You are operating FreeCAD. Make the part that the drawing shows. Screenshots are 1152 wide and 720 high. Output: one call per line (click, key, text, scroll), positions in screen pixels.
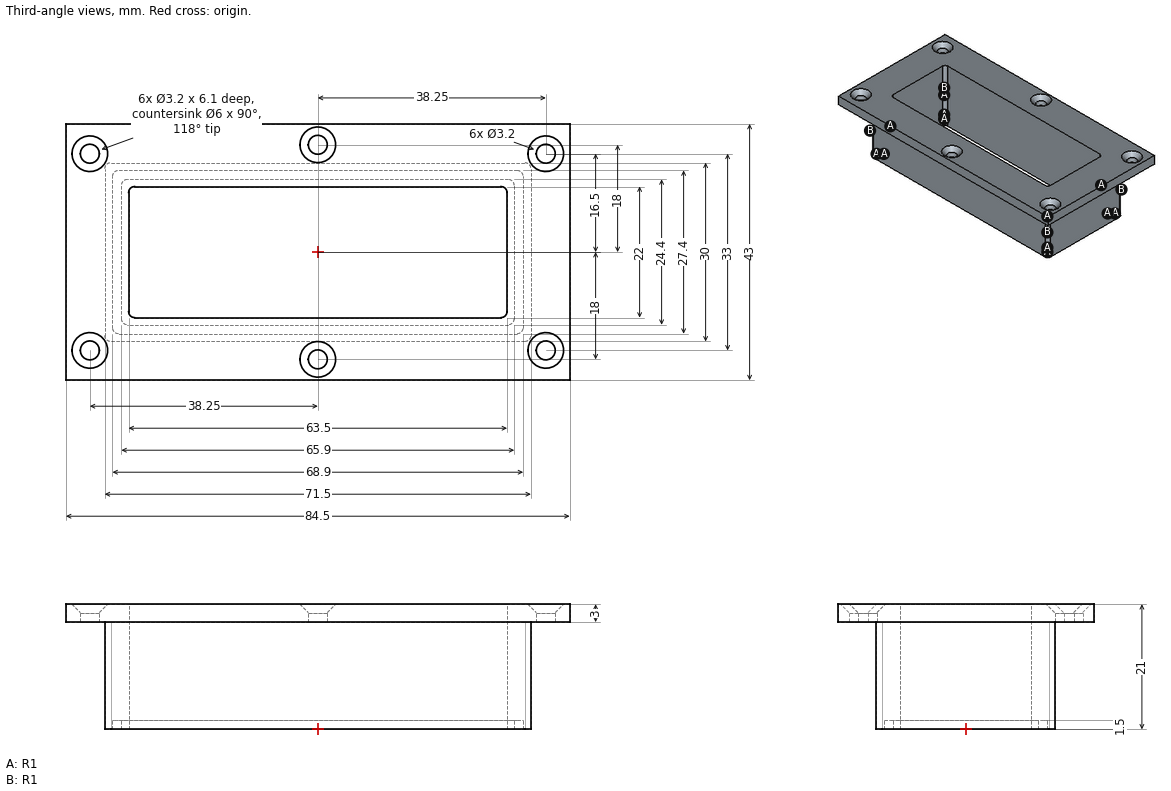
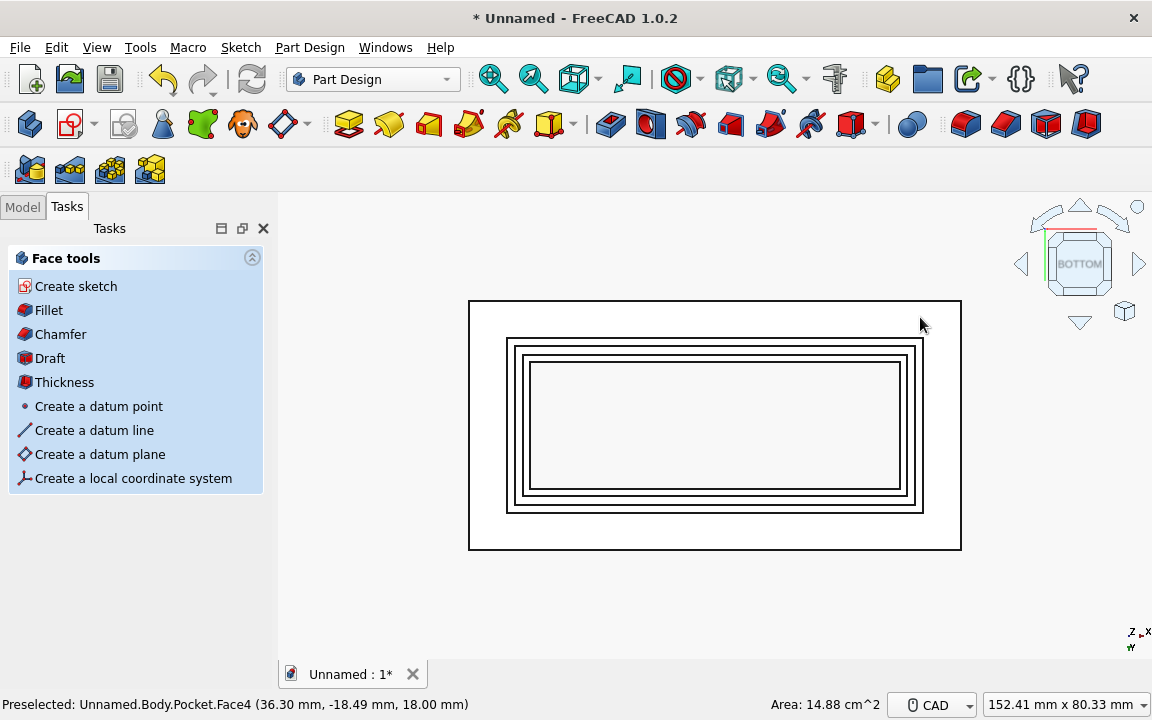
click(70, 124)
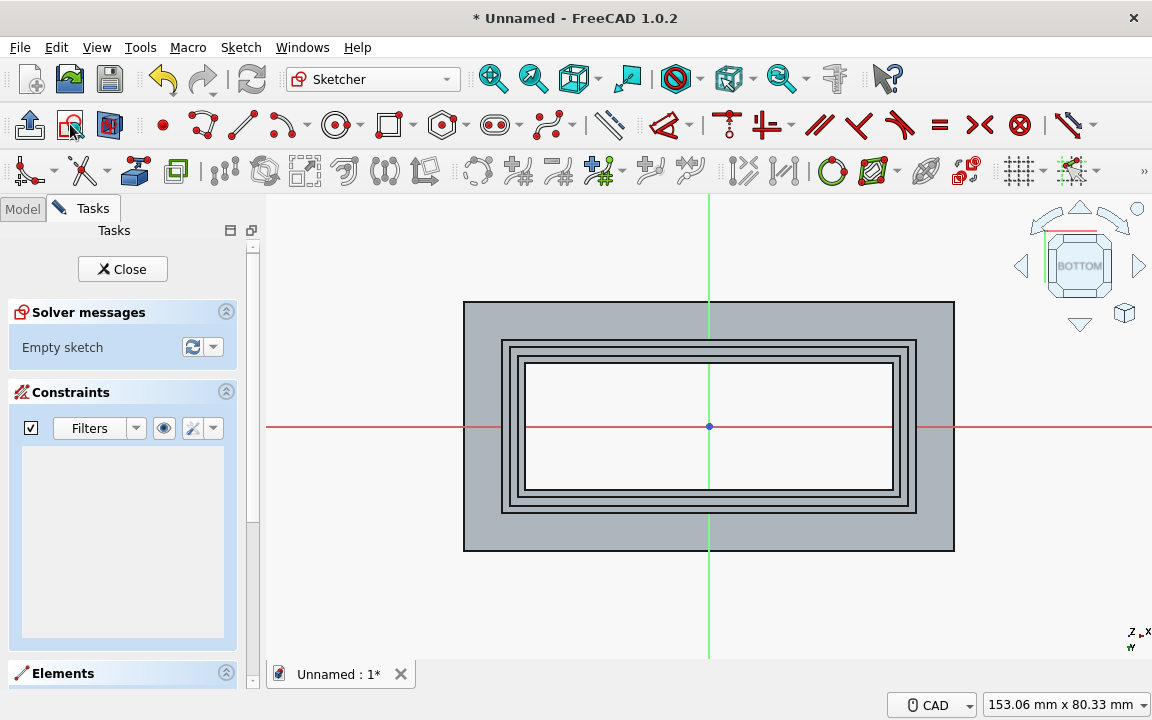
click(336, 126)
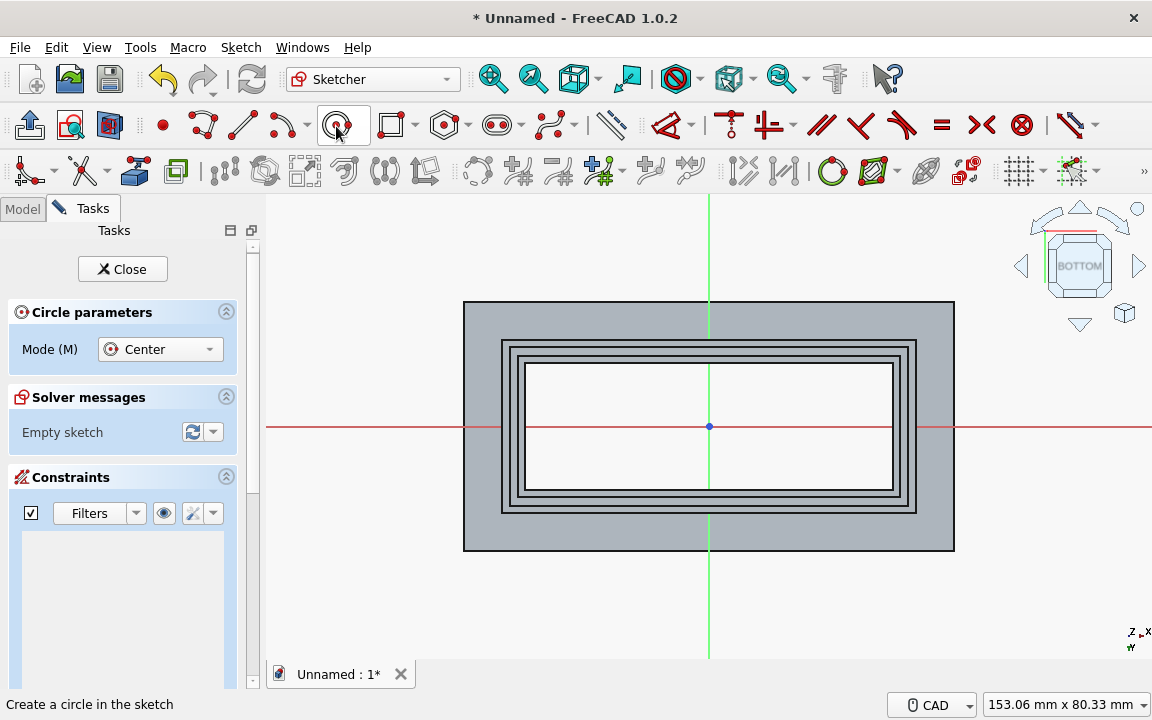
scroll(930, 522, up, 5)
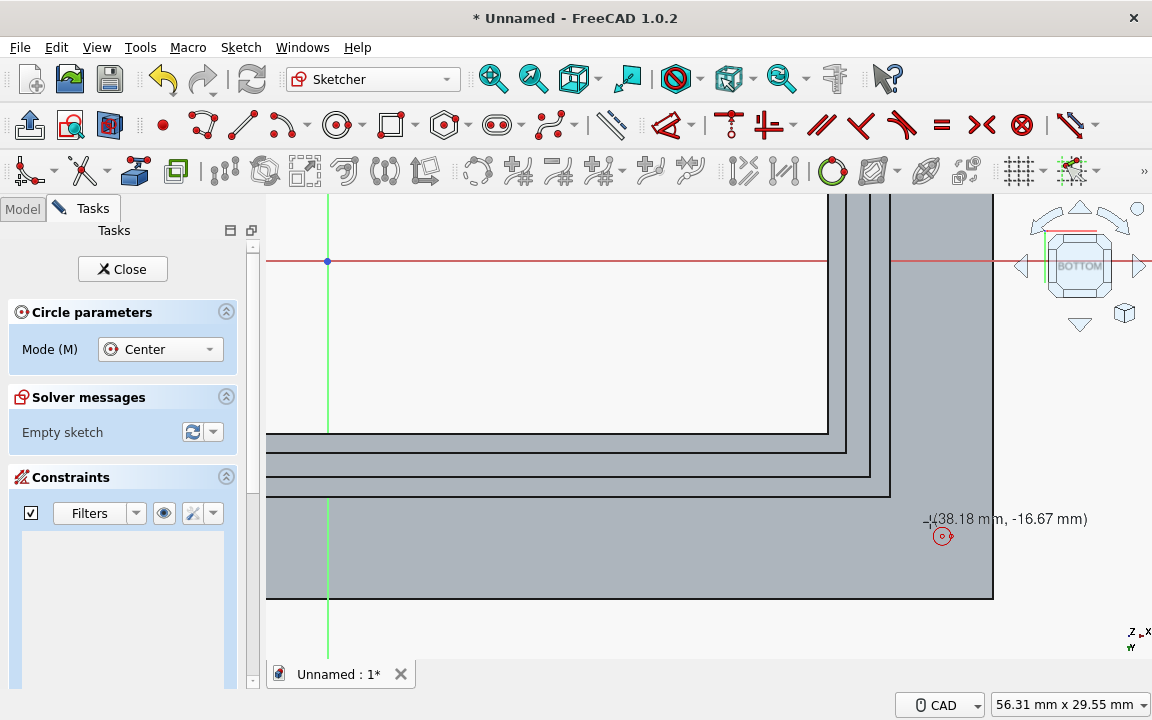
click(930, 521)
click(948, 503)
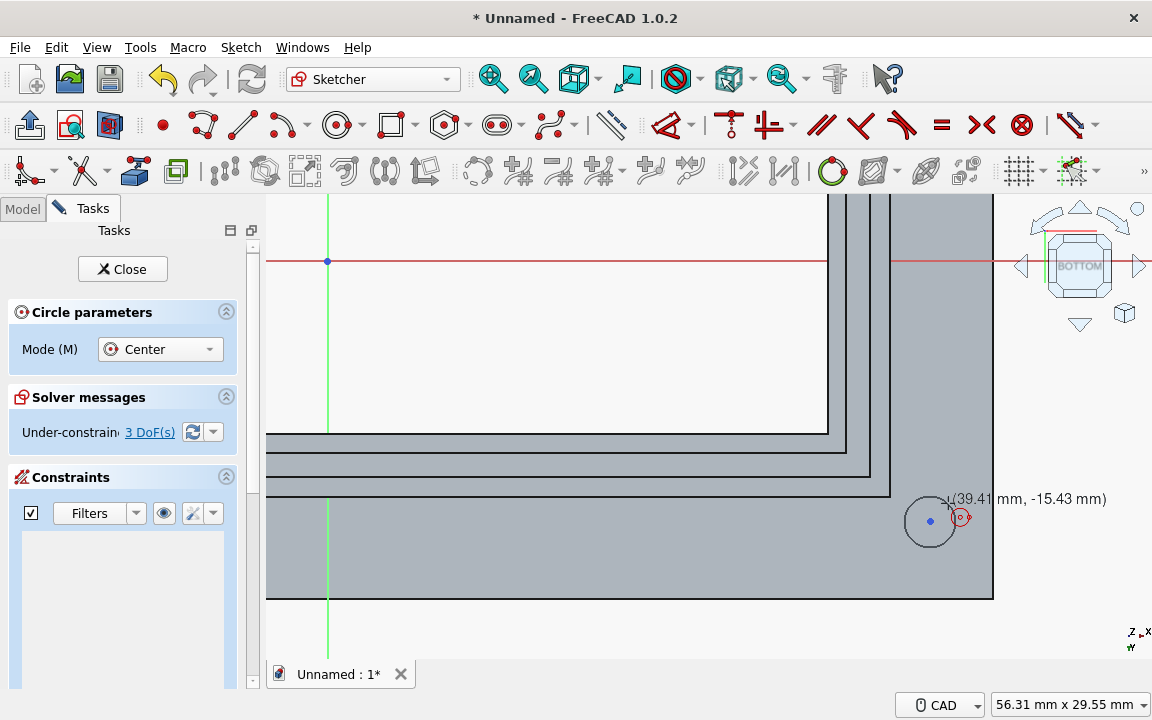
scroll(822, 523, down, 5)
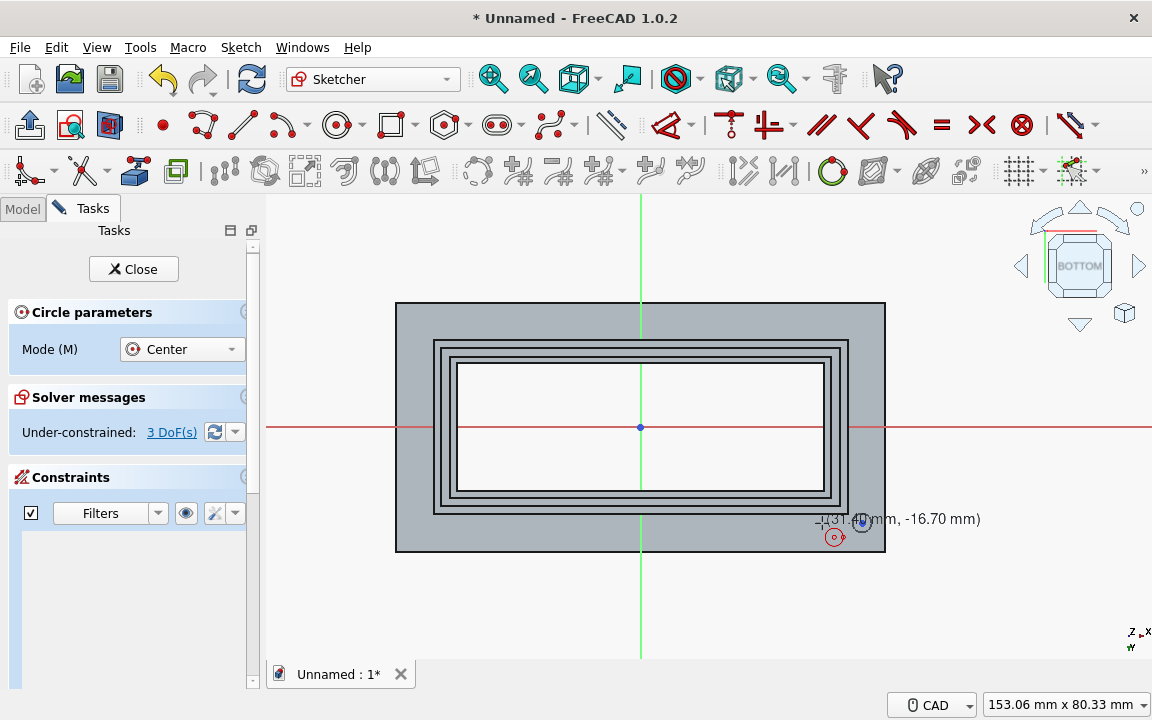
scroll(862, 332, up, 5)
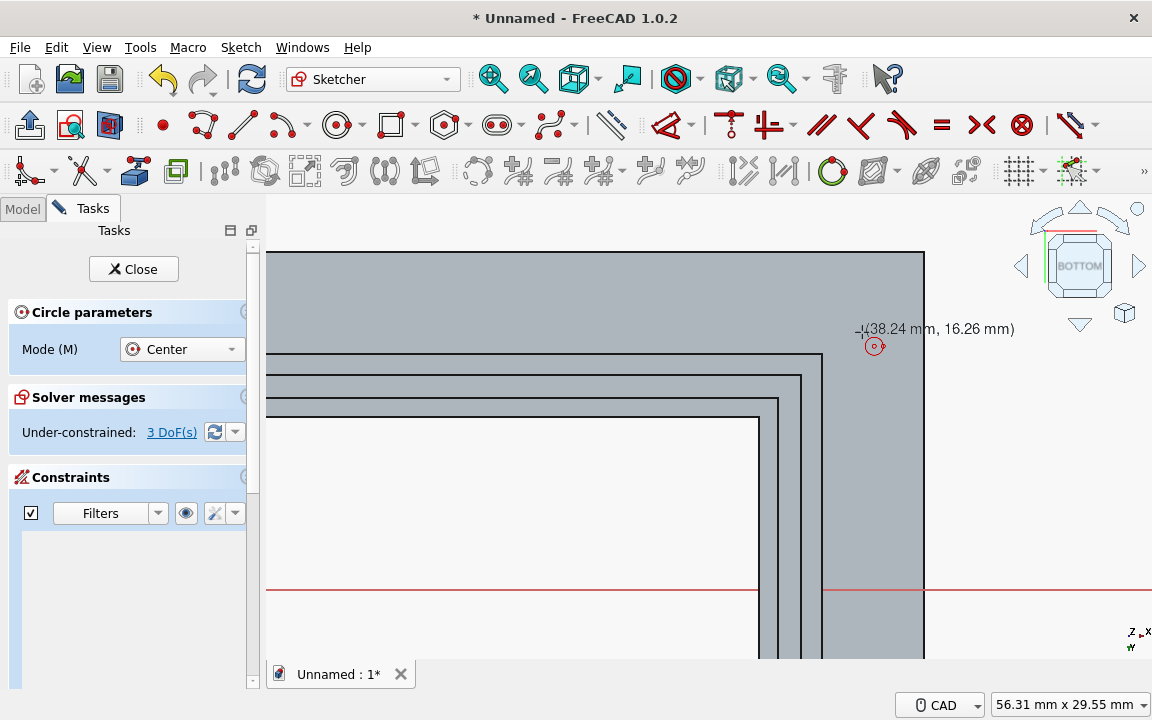
click(861, 330)
click(879, 313)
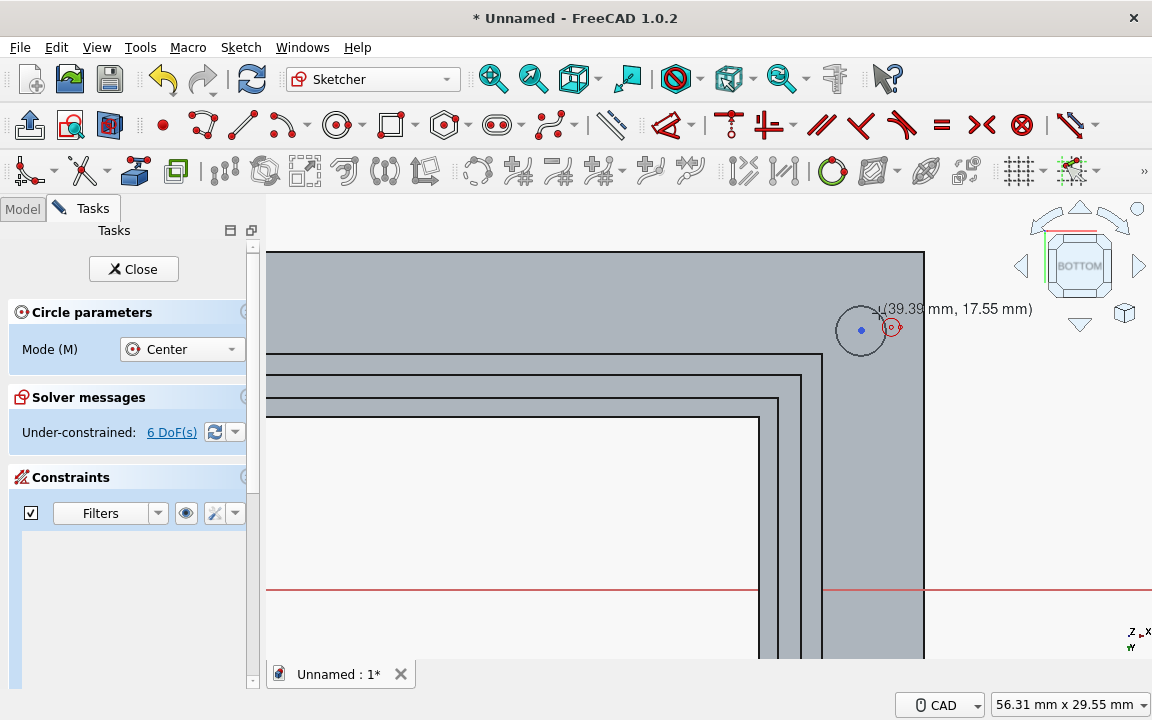
scroll(862, 331, down, 5)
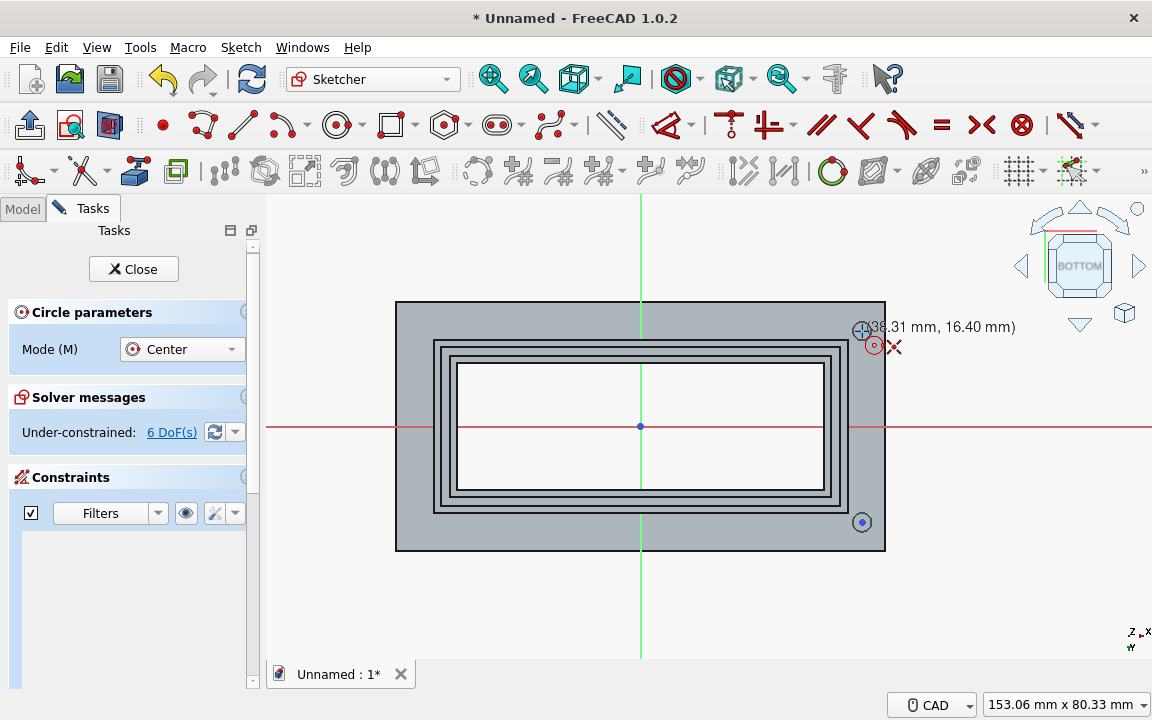
scroll(419, 331, up, 5)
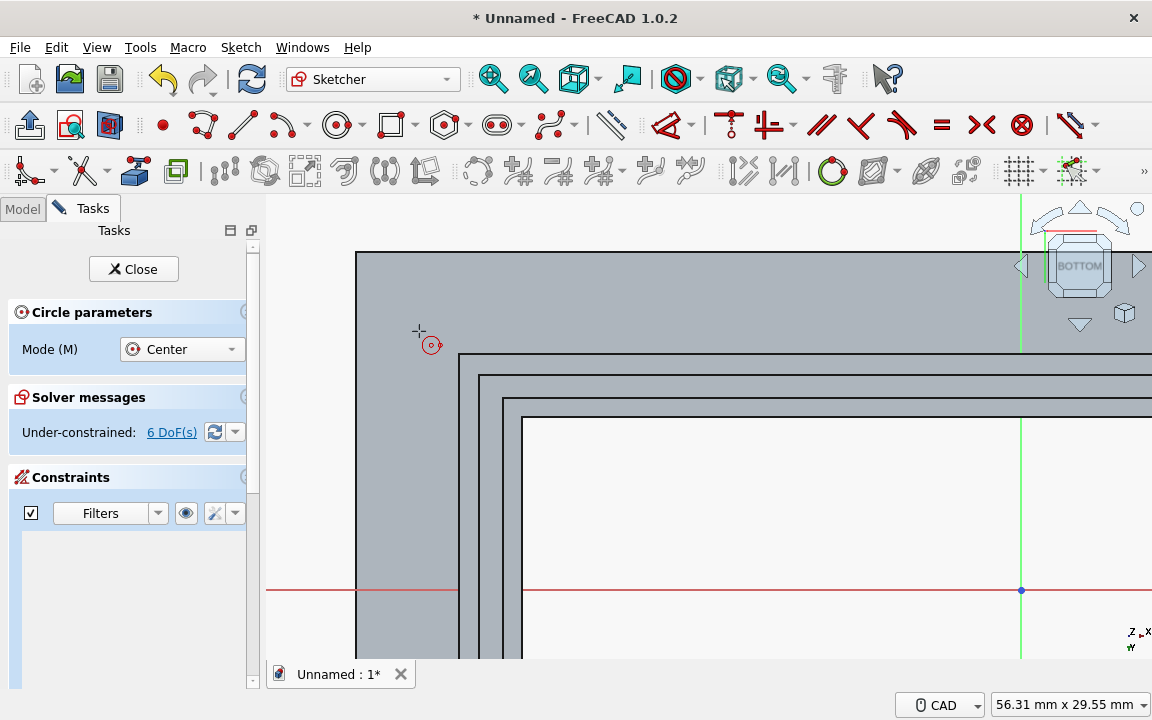
click(419, 330)
click(437, 313)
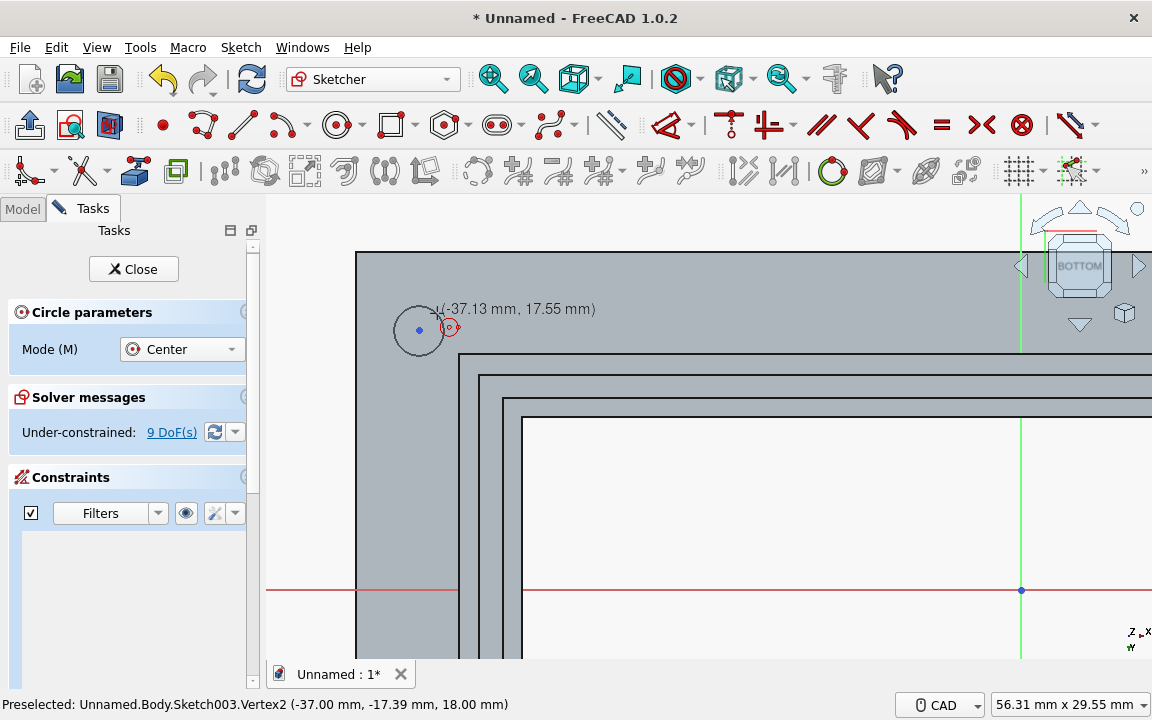
scroll(419, 331, down, 5)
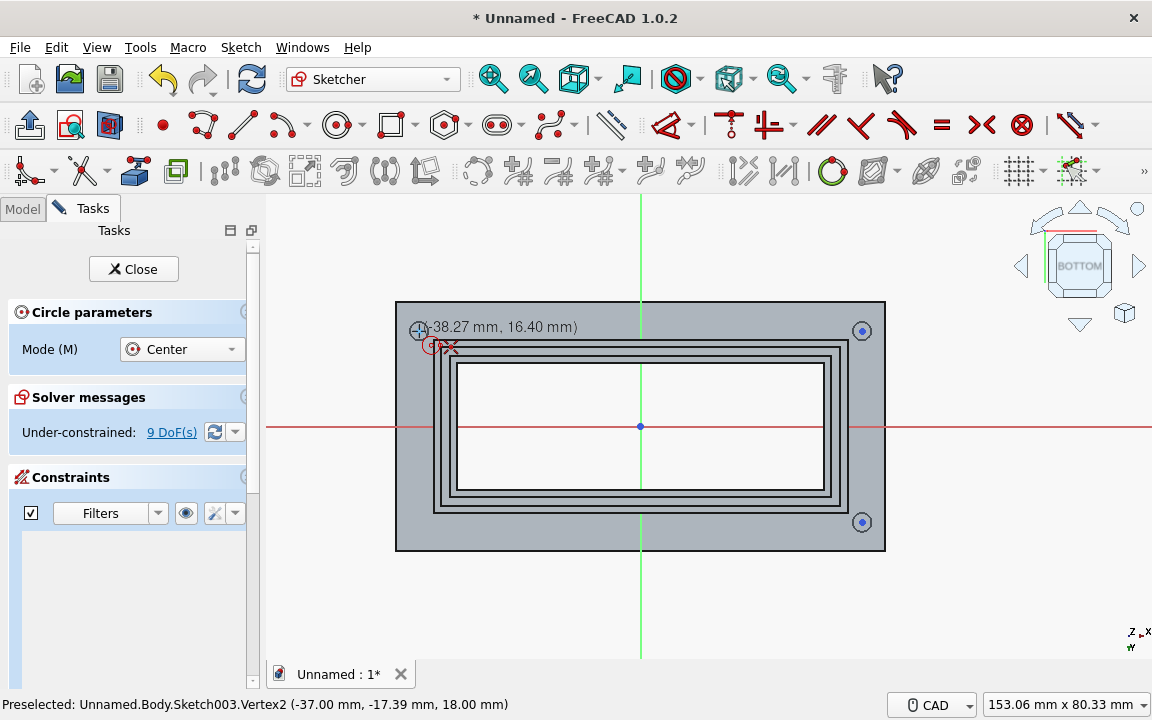
scroll(419, 522, up, 5)